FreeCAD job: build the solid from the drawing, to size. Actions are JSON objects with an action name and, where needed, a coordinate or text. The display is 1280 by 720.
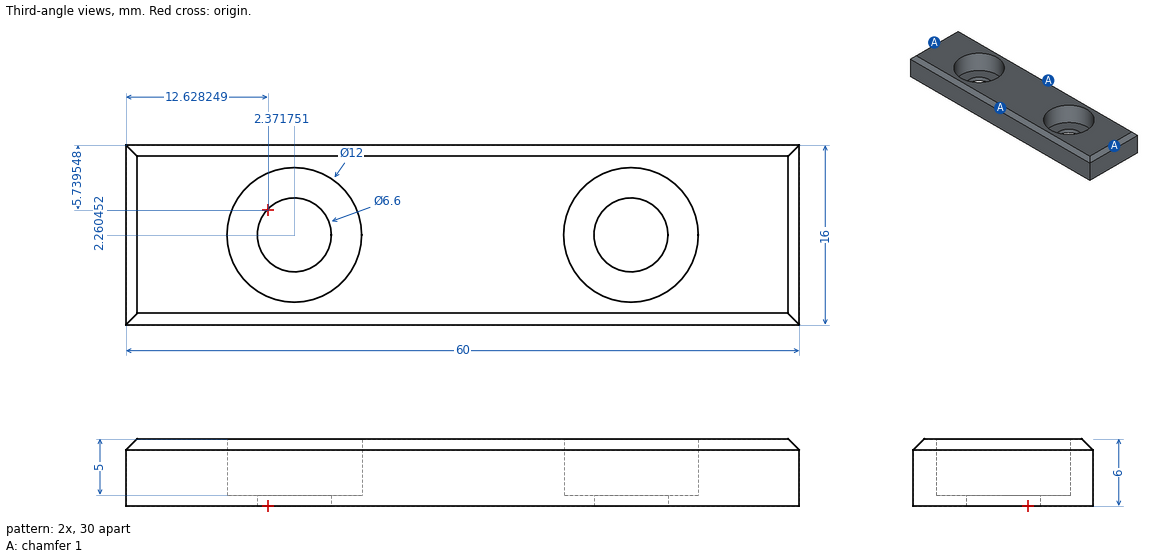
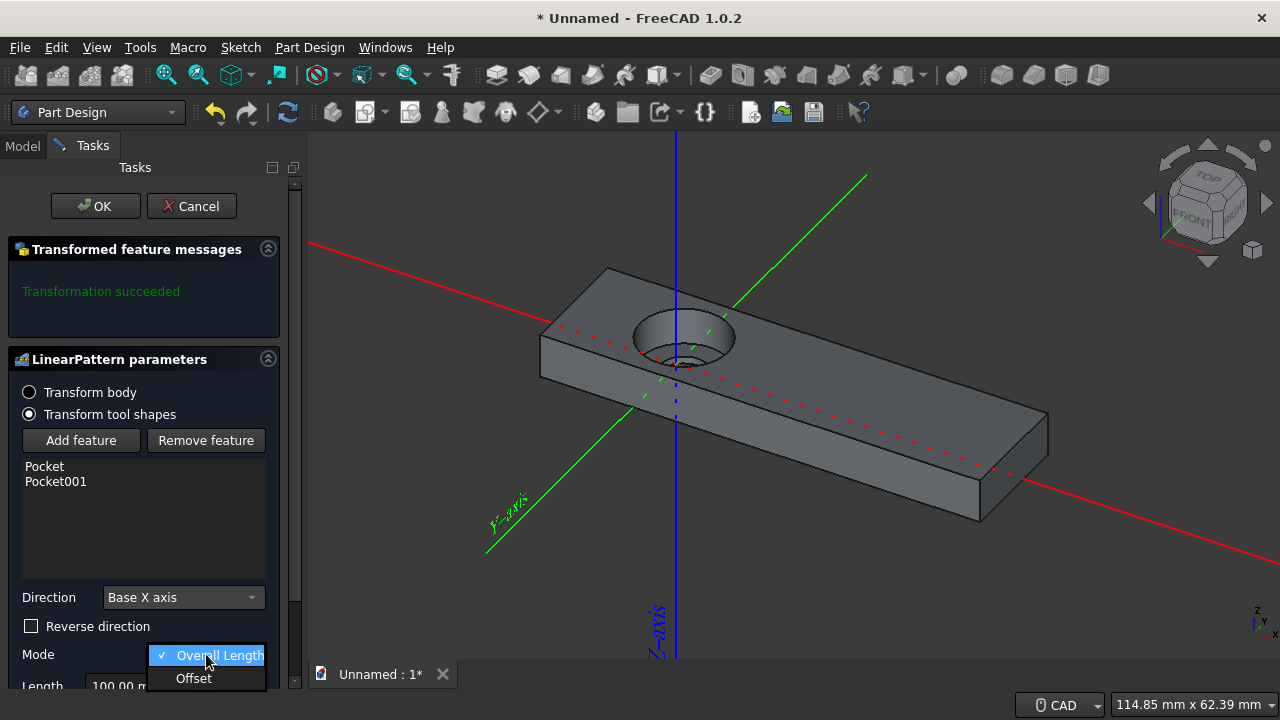
{"action": "left_click", "coordinate": [206, 678]}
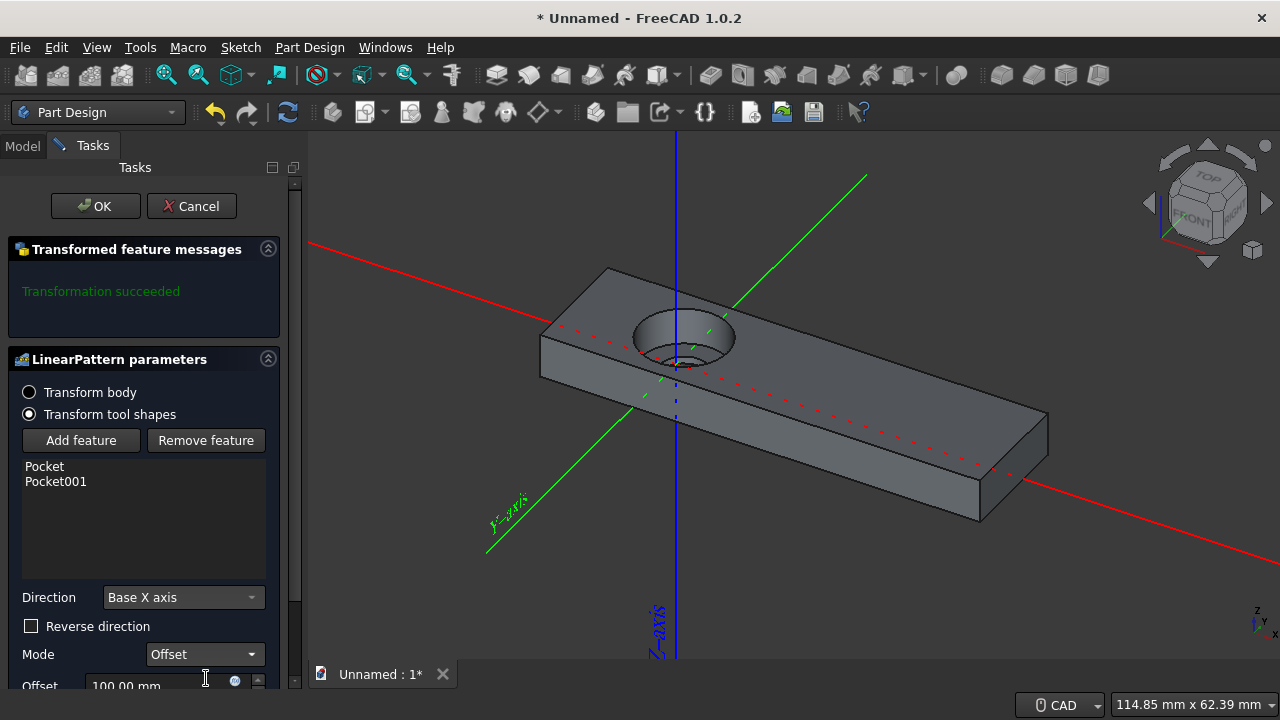
{"action": "scroll", "coordinate": [295, 432], "scroll_direction": "down", "scroll_amount": 2}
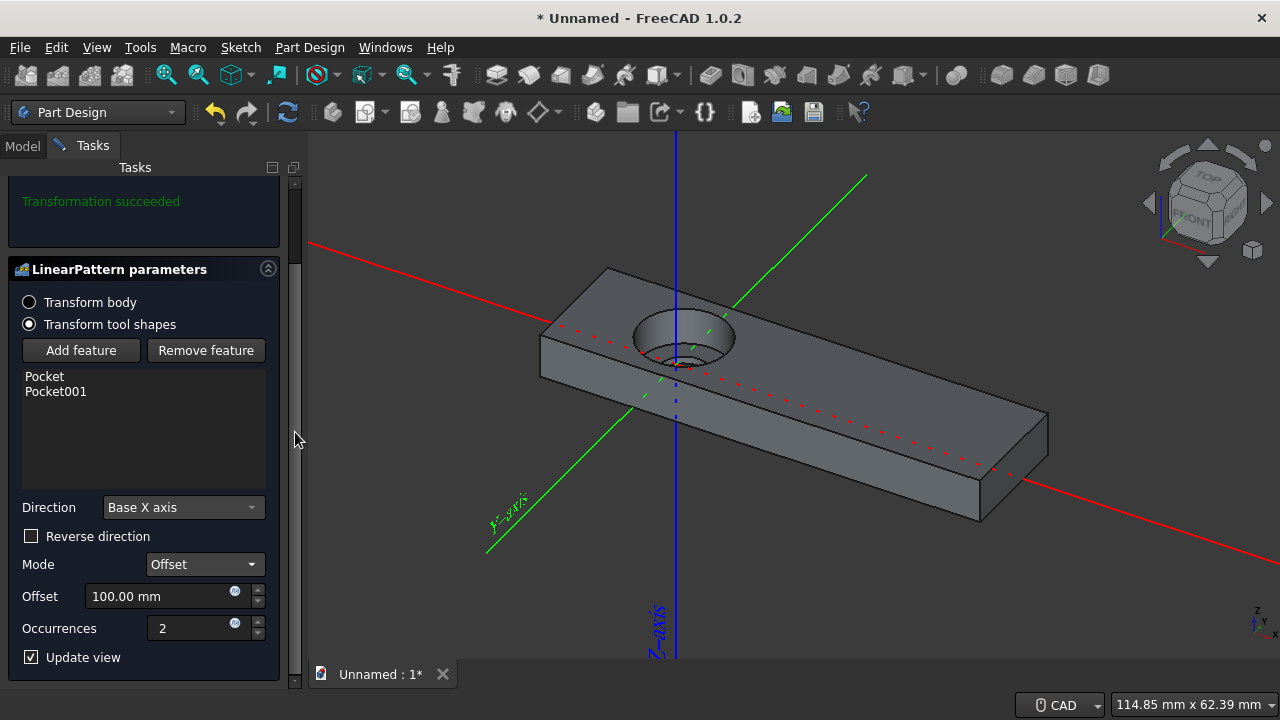
{"action": "triple_click", "coordinate": [168, 596]}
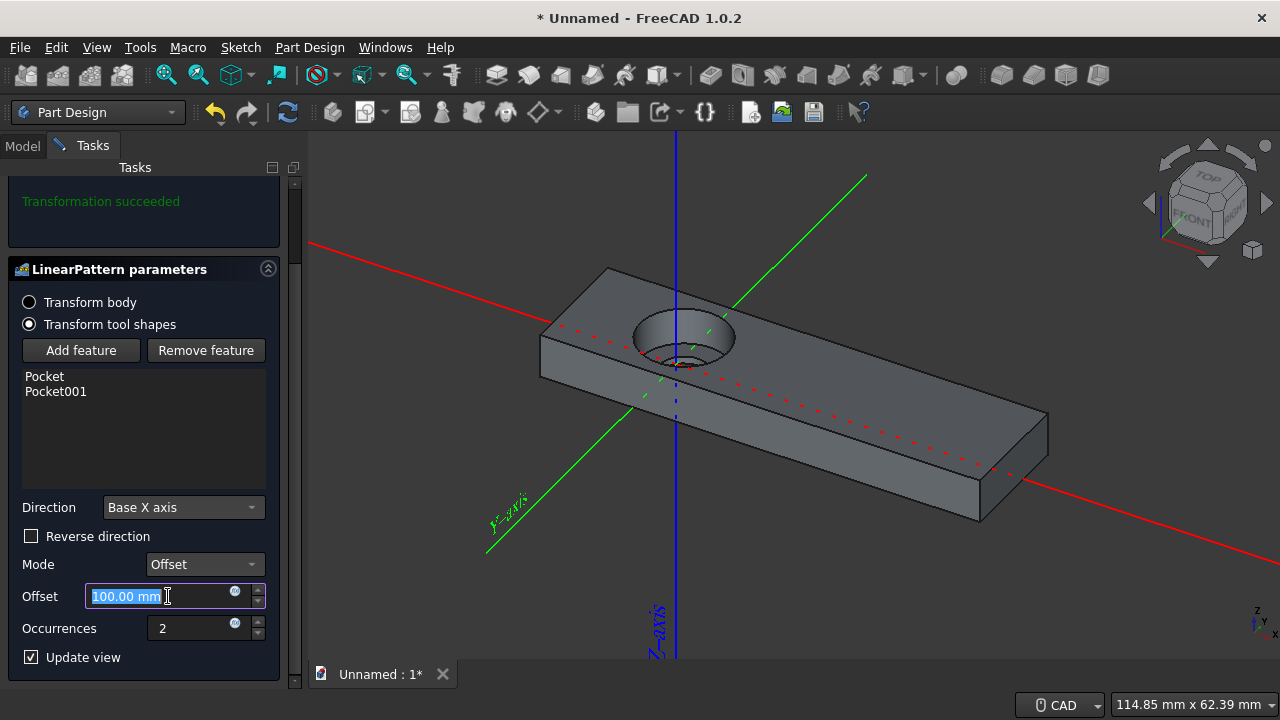
{"action": "type", "text": "30"}
{"action": "key", "text": "Tab"}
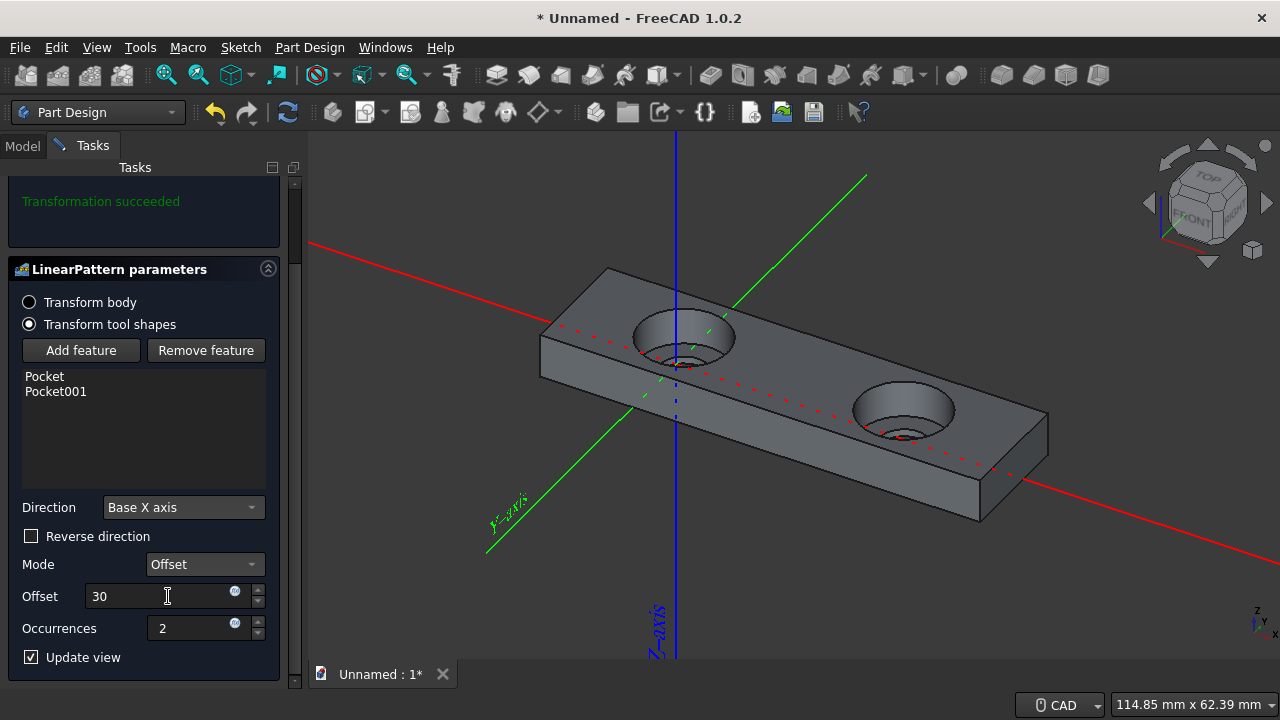
{"action": "triple_click", "coordinate": [198, 628]}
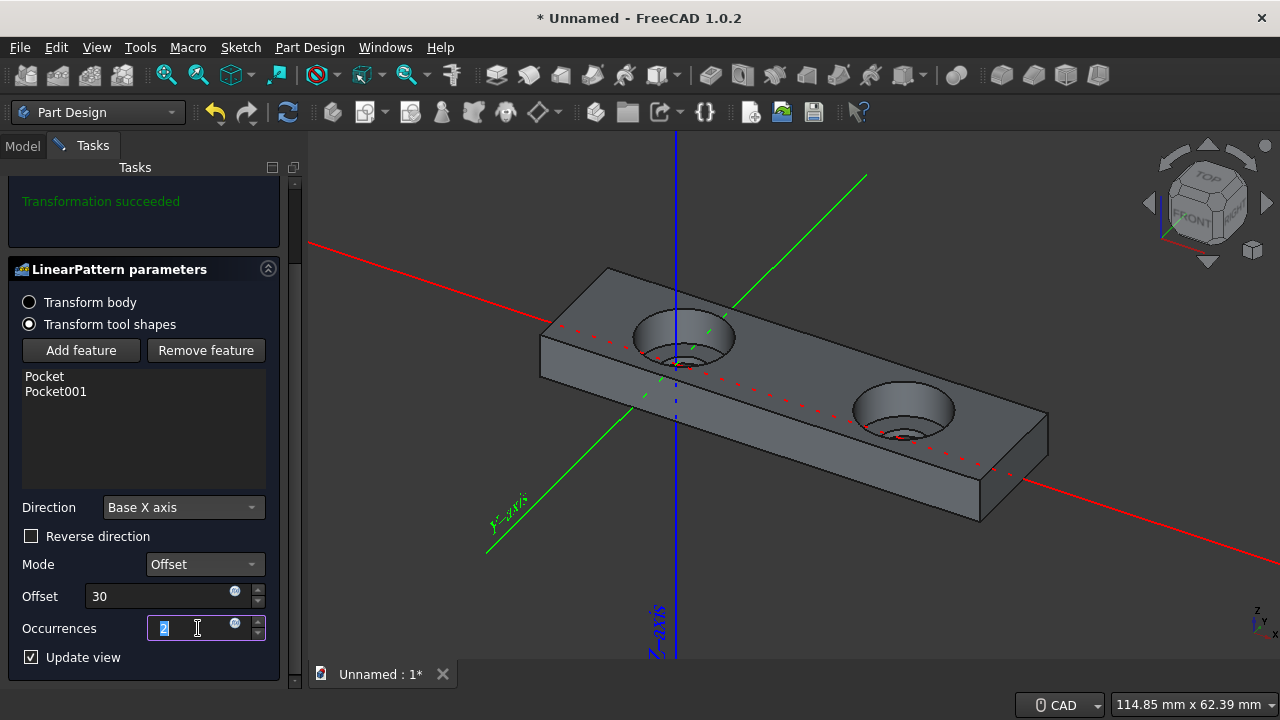
{"action": "type", "text": "2"}
{"action": "key", "text": "Tab"}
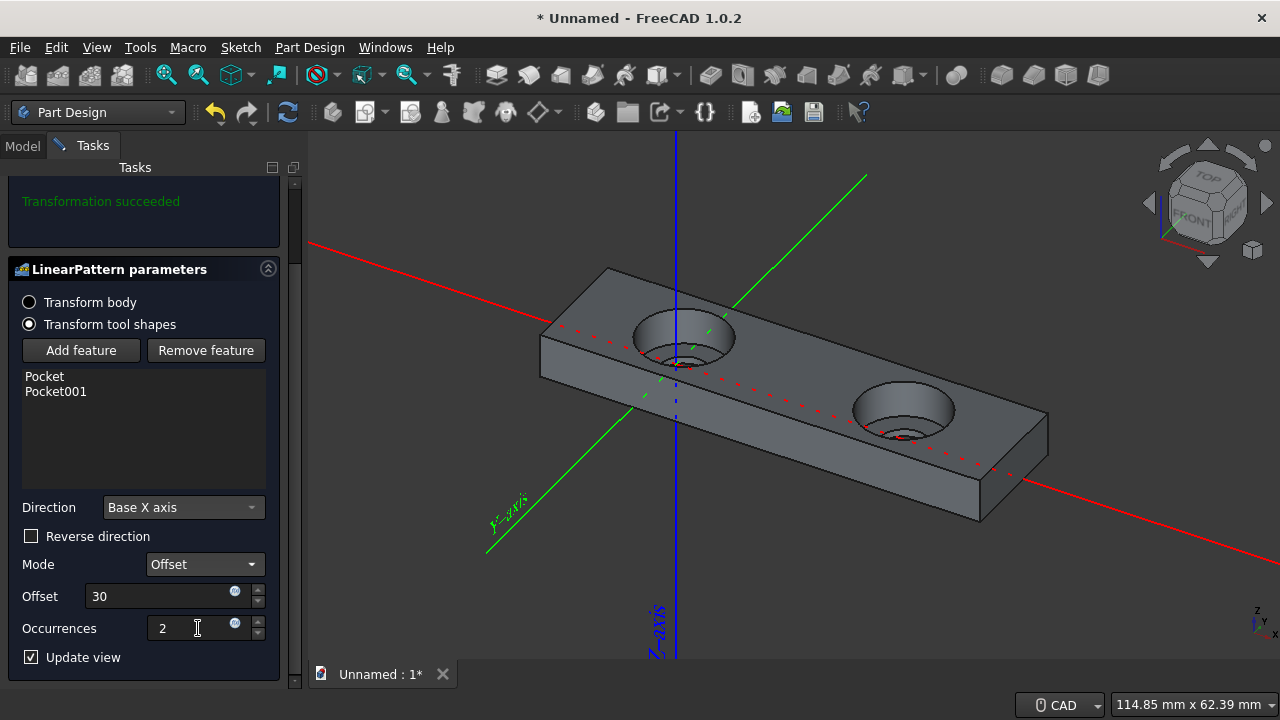
{"action": "scroll", "coordinate": [295, 432], "scroll_direction": "up", "scroll_amount": 3}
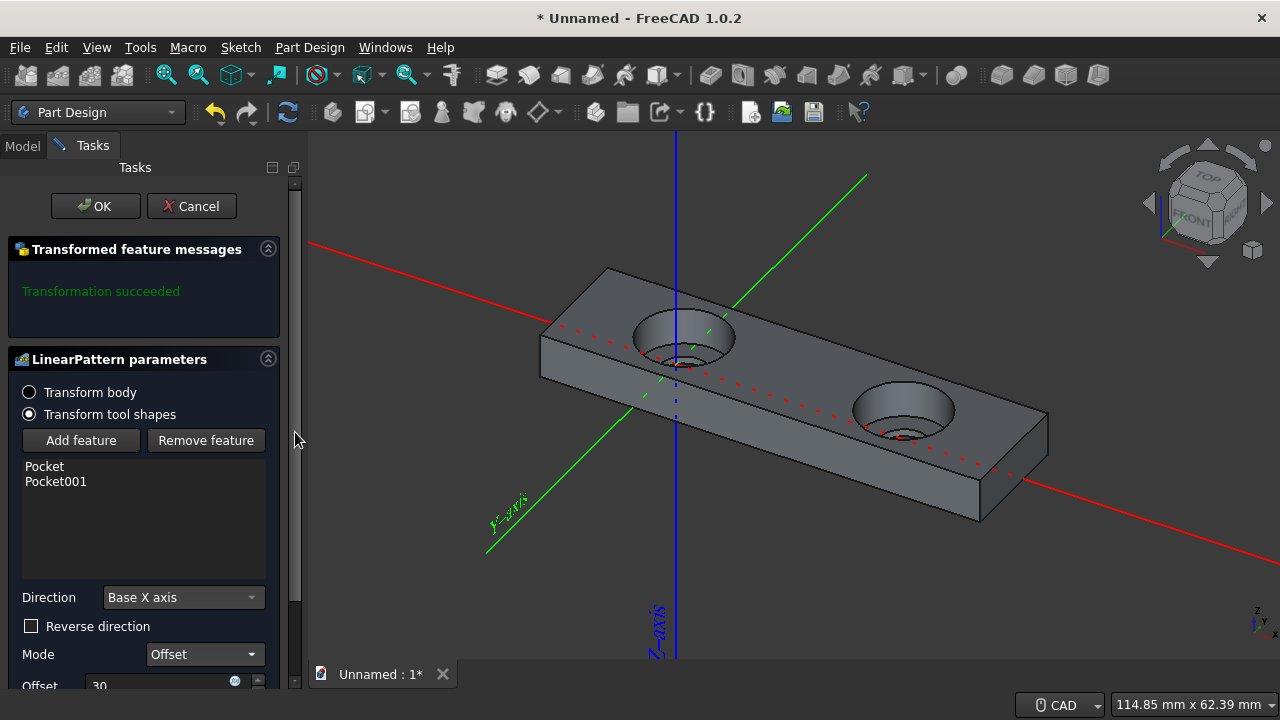
{"action": "left_click", "coordinate": [96, 206]}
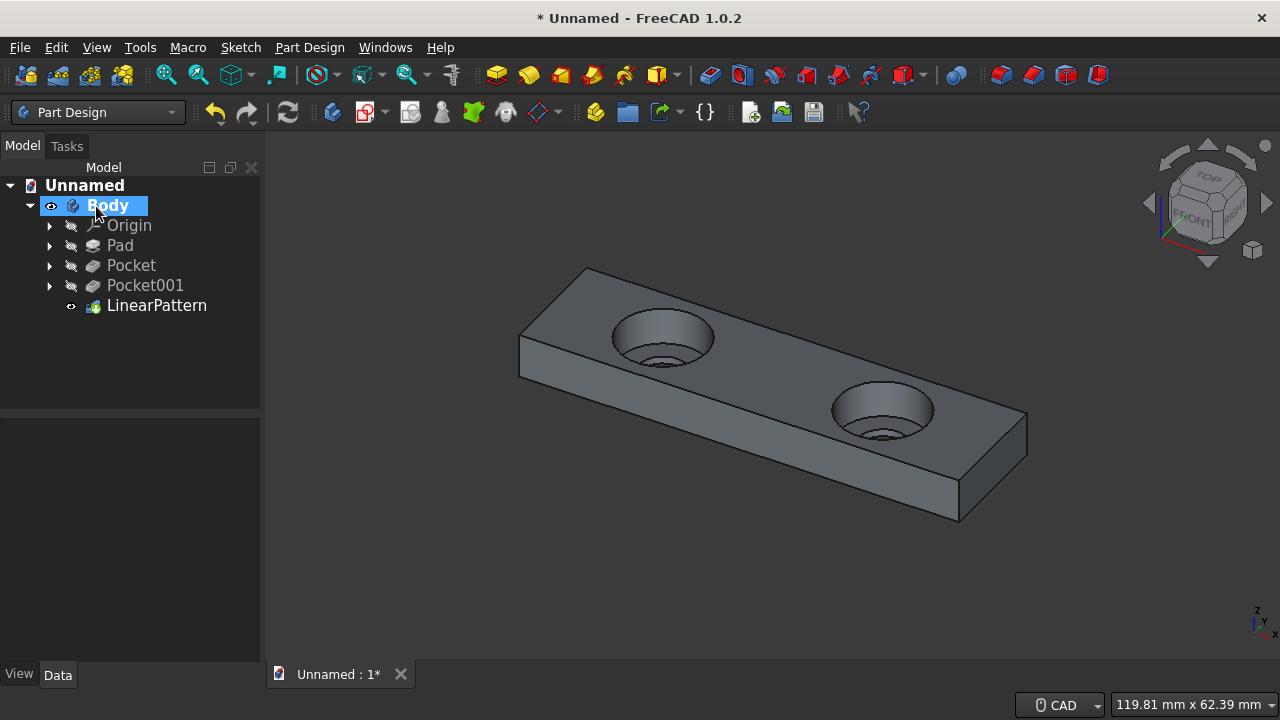
{"action": "left_click", "coordinate": [993, 446]}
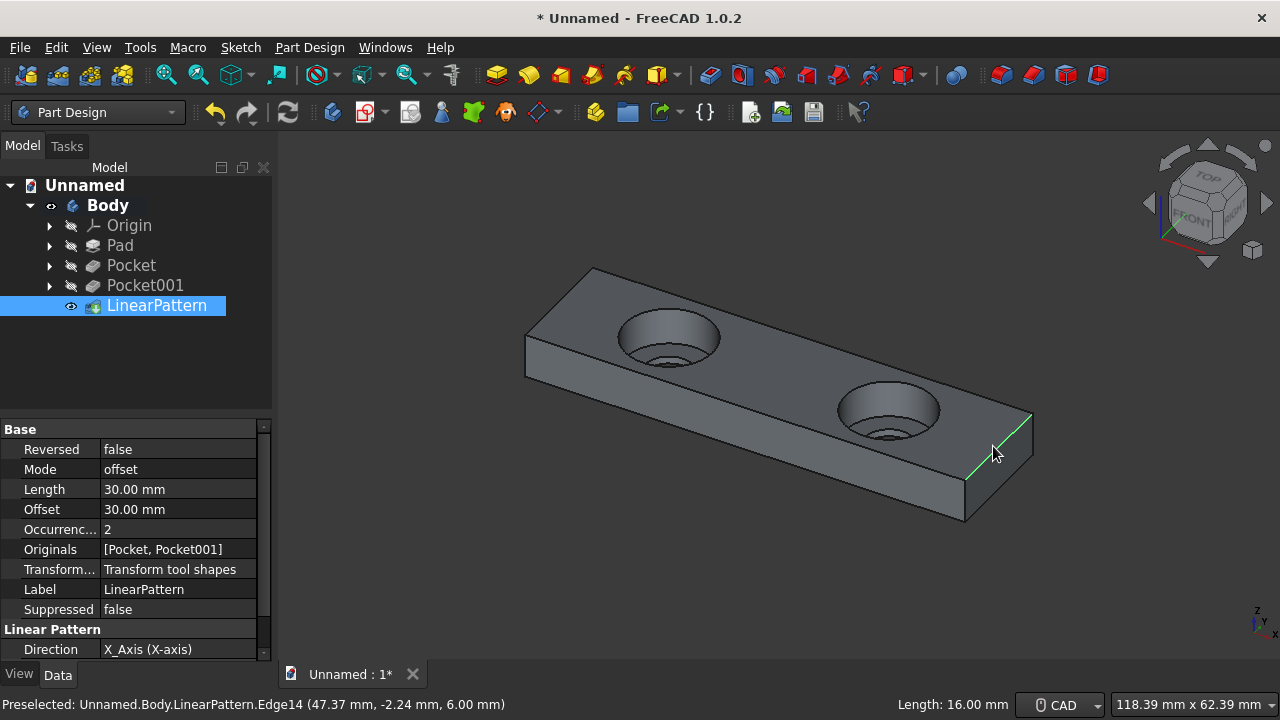
{"action": "left_click", "coordinate": [745, 407], "text": "ctrl"}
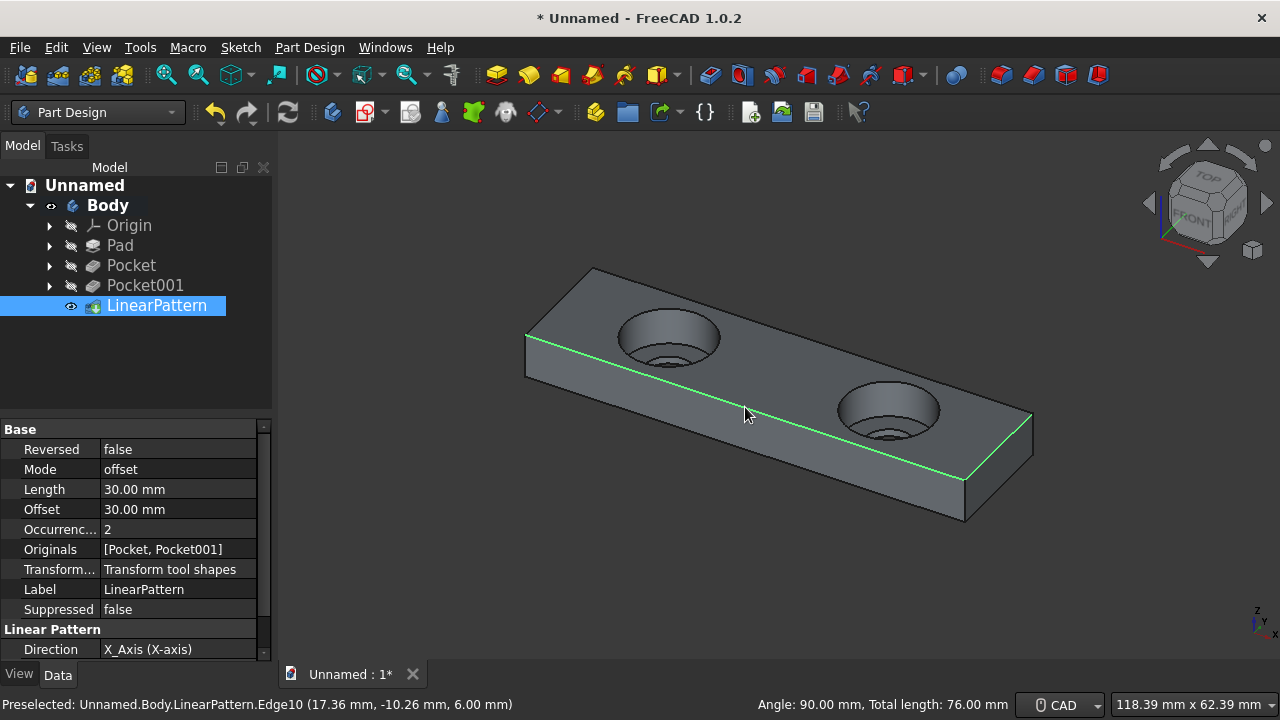
{"action": "key", "text": "0"}